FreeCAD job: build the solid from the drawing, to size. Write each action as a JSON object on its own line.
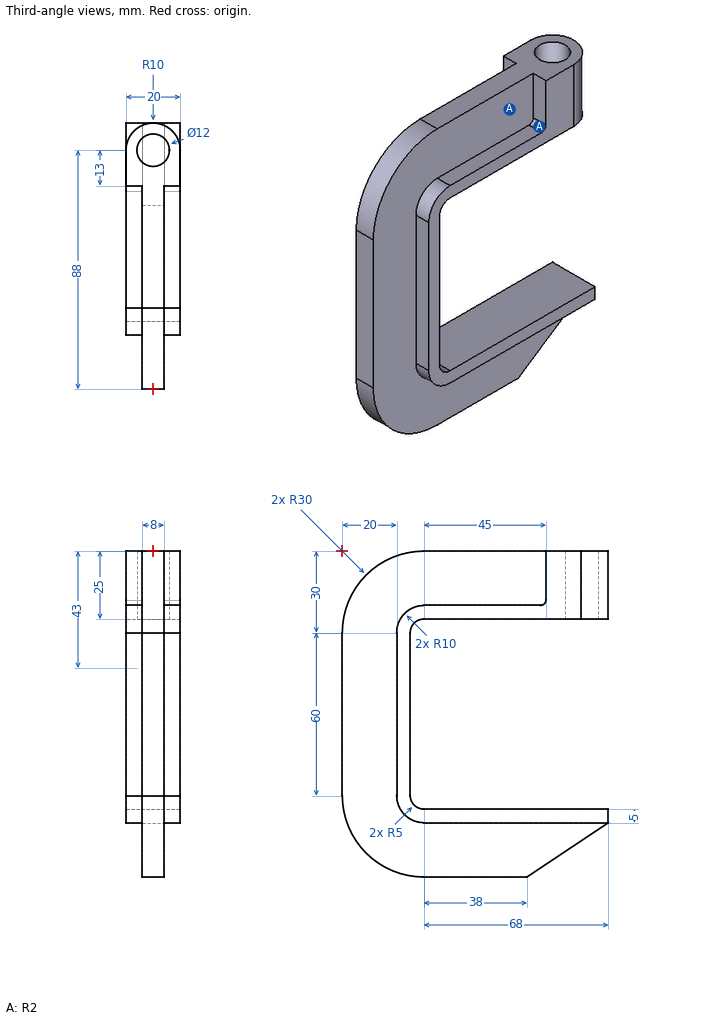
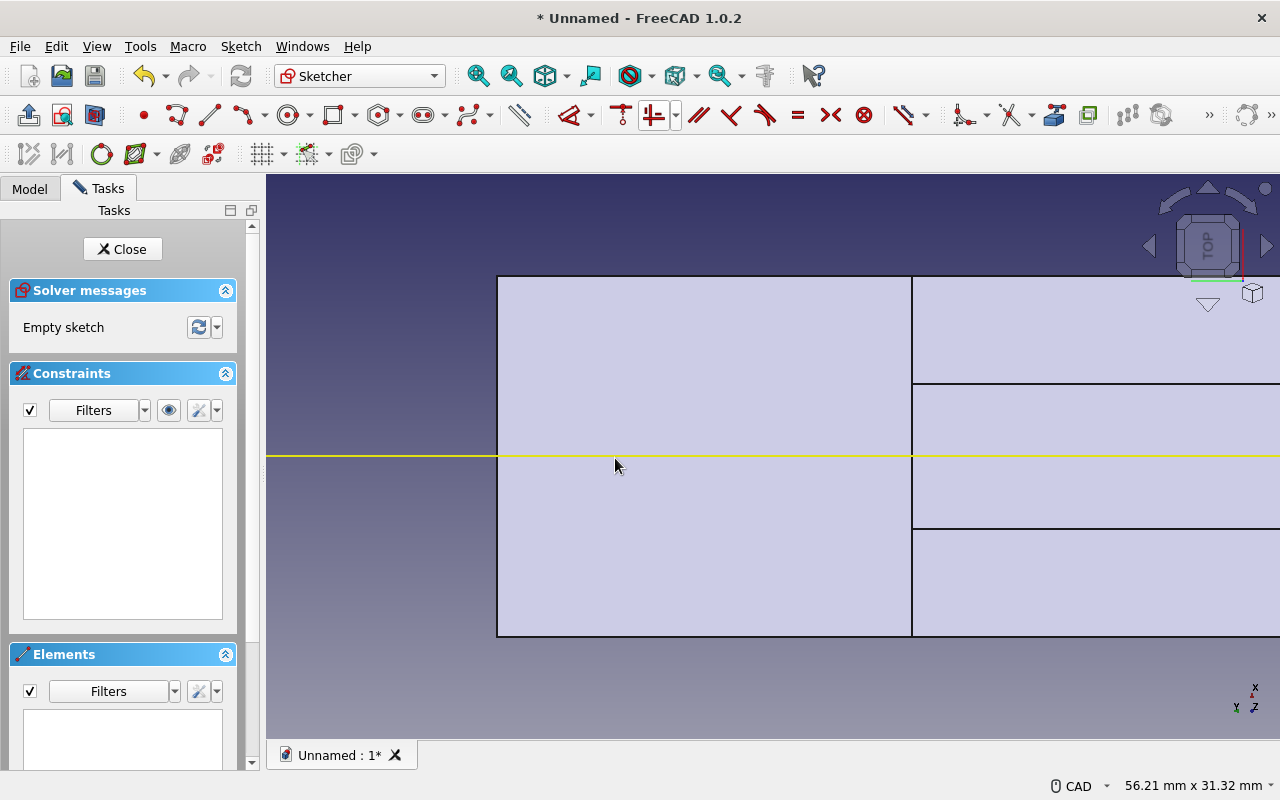
{"action": "key", "text": "g m"}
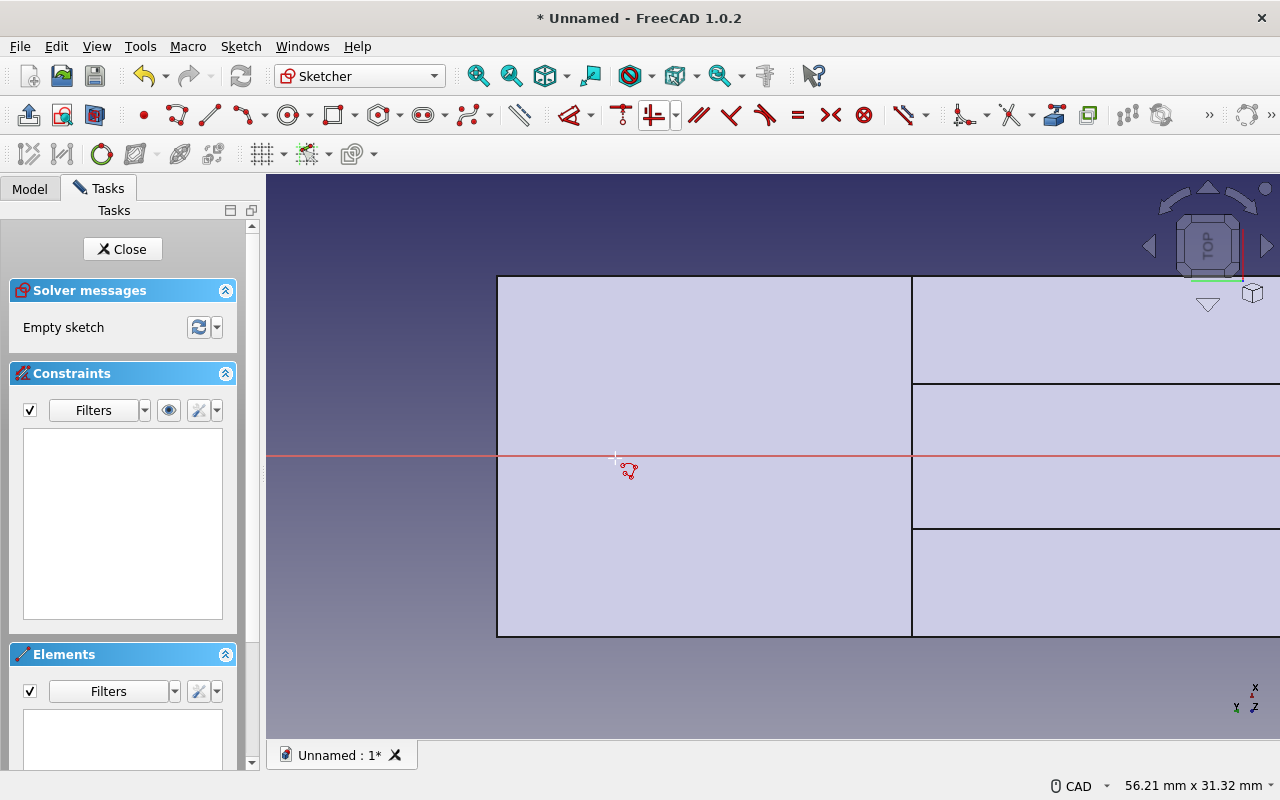
{"action": "left_click", "coordinate": [677, 637]}
{"action": "left_click", "coordinate": [912, 637]}
{"action": "left_click", "coordinate": [912, 276]}
{"action": "left_click", "coordinate": [677, 276]}
{"action": "right_click", "coordinate": [677, 276]}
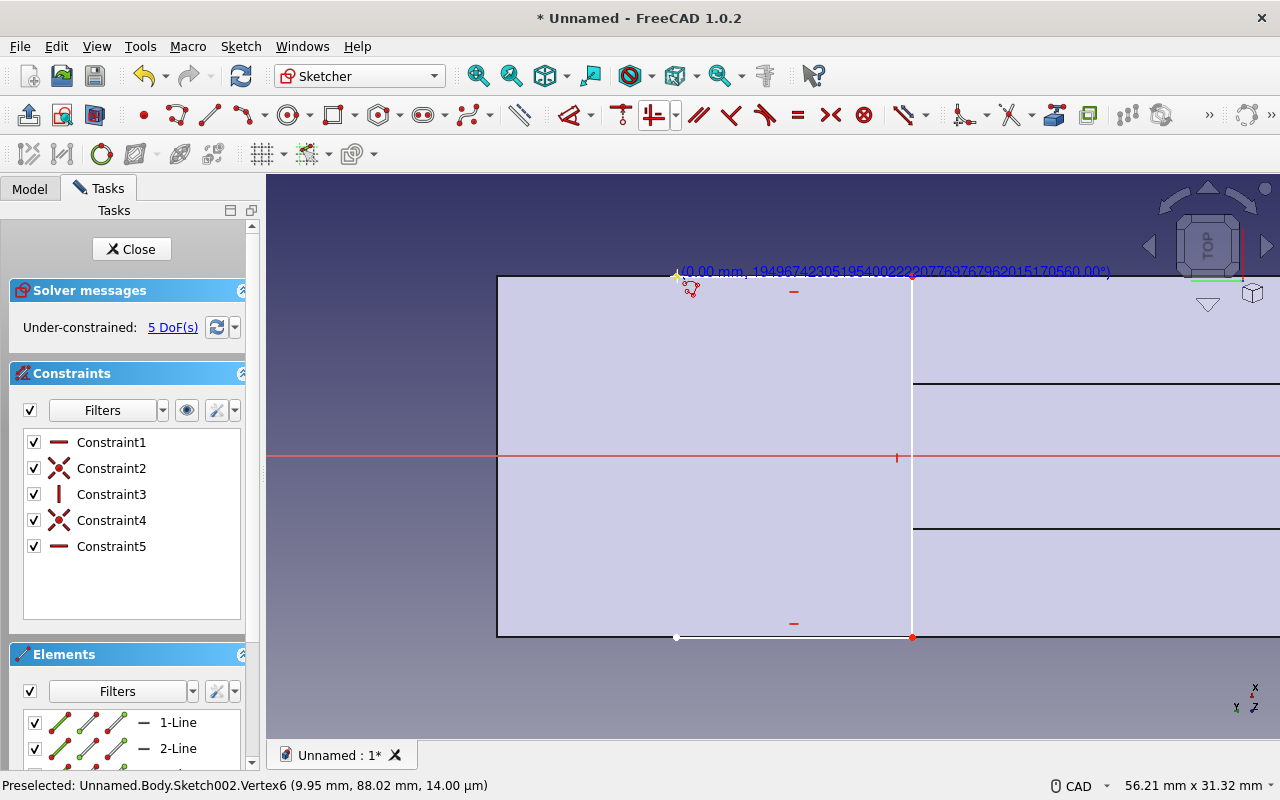
{"action": "key", "text": "g 3 a"}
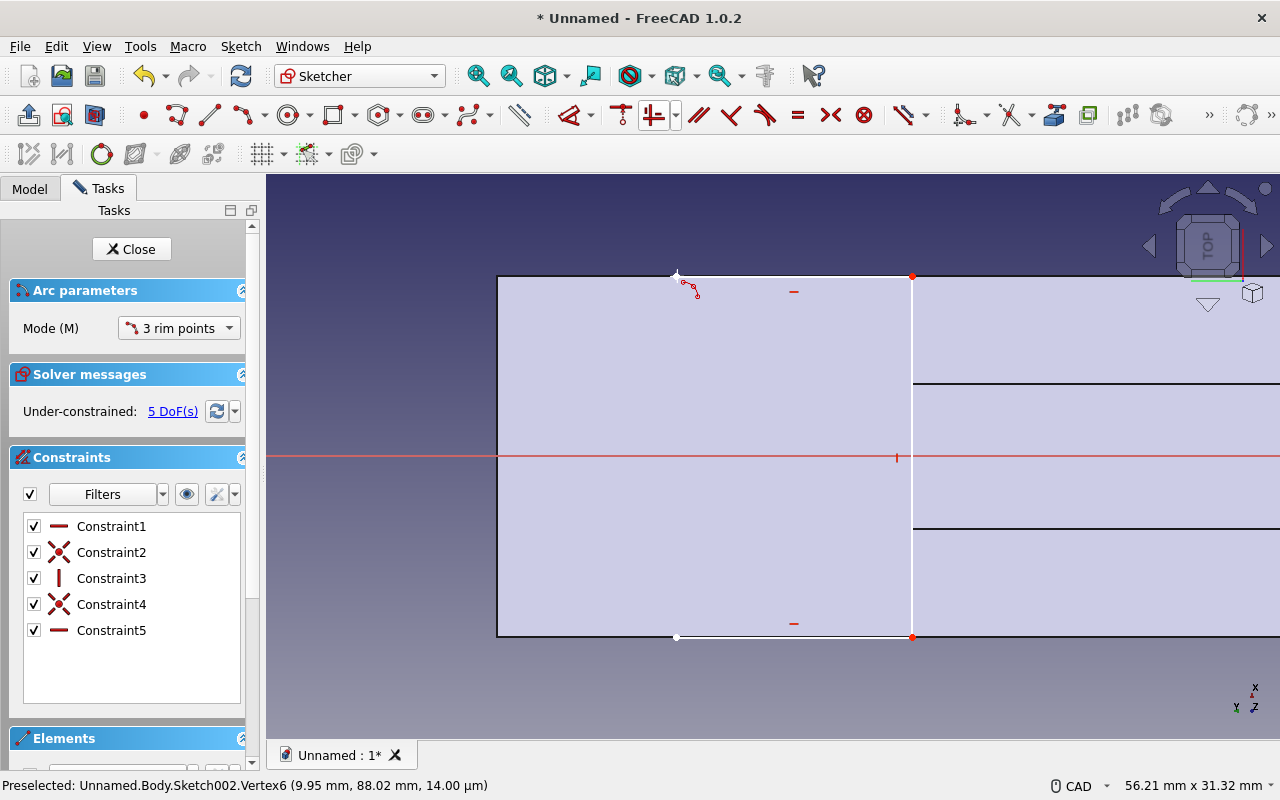
{"action": "left_click", "coordinate": [677, 277]}
{"action": "left_click", "coordinate": [677, 638]}
{"action": "left_click", "coordinate": [506, 401]}
{"action": "key", "text": "Escape"}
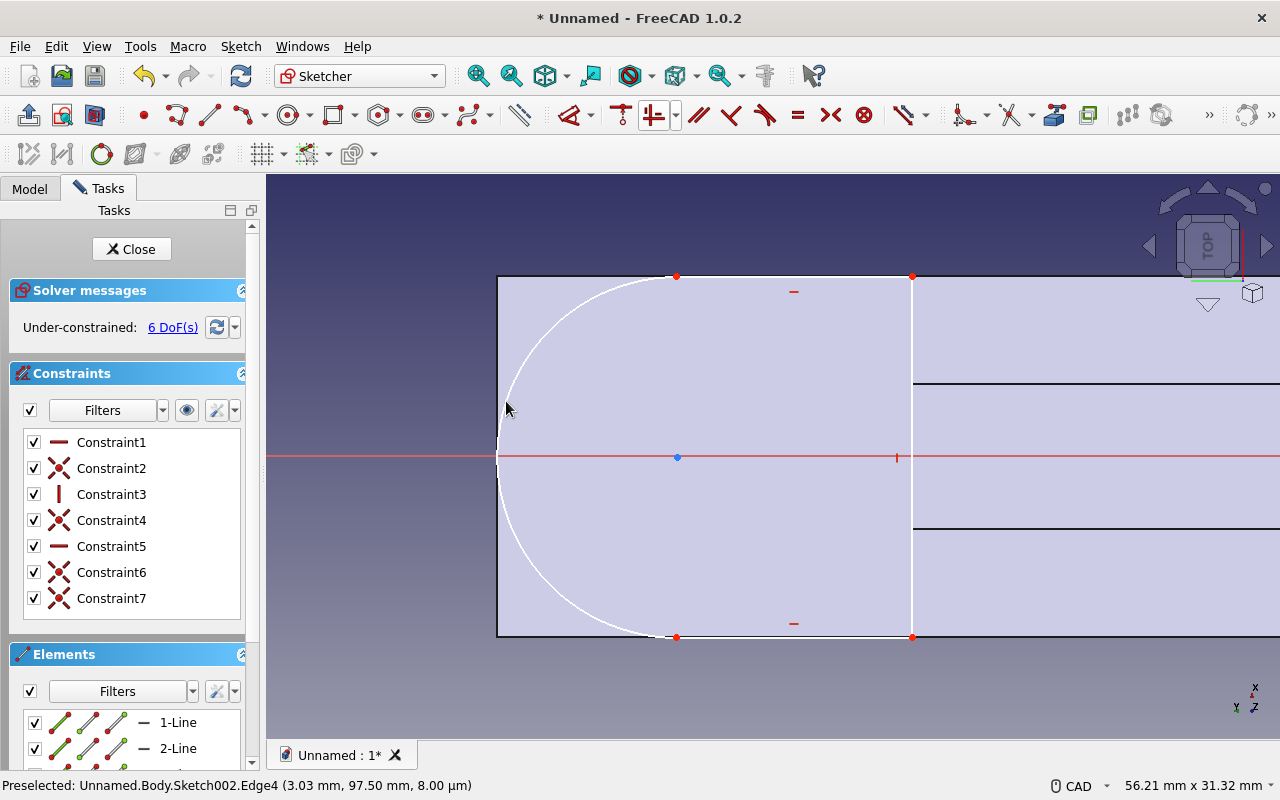
{"action": "left_click", "coordinate": [748, 638]}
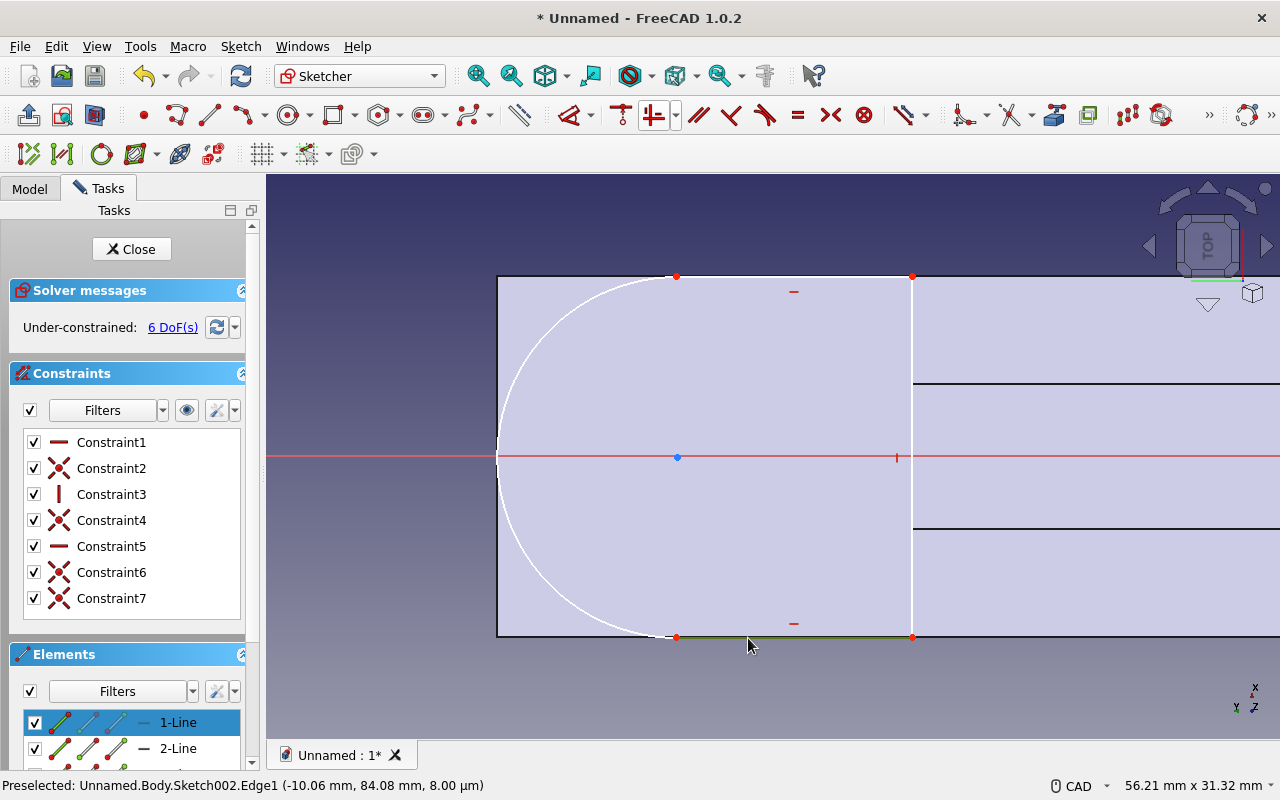
{"action": "left_click", "coordinate": [532, 352]}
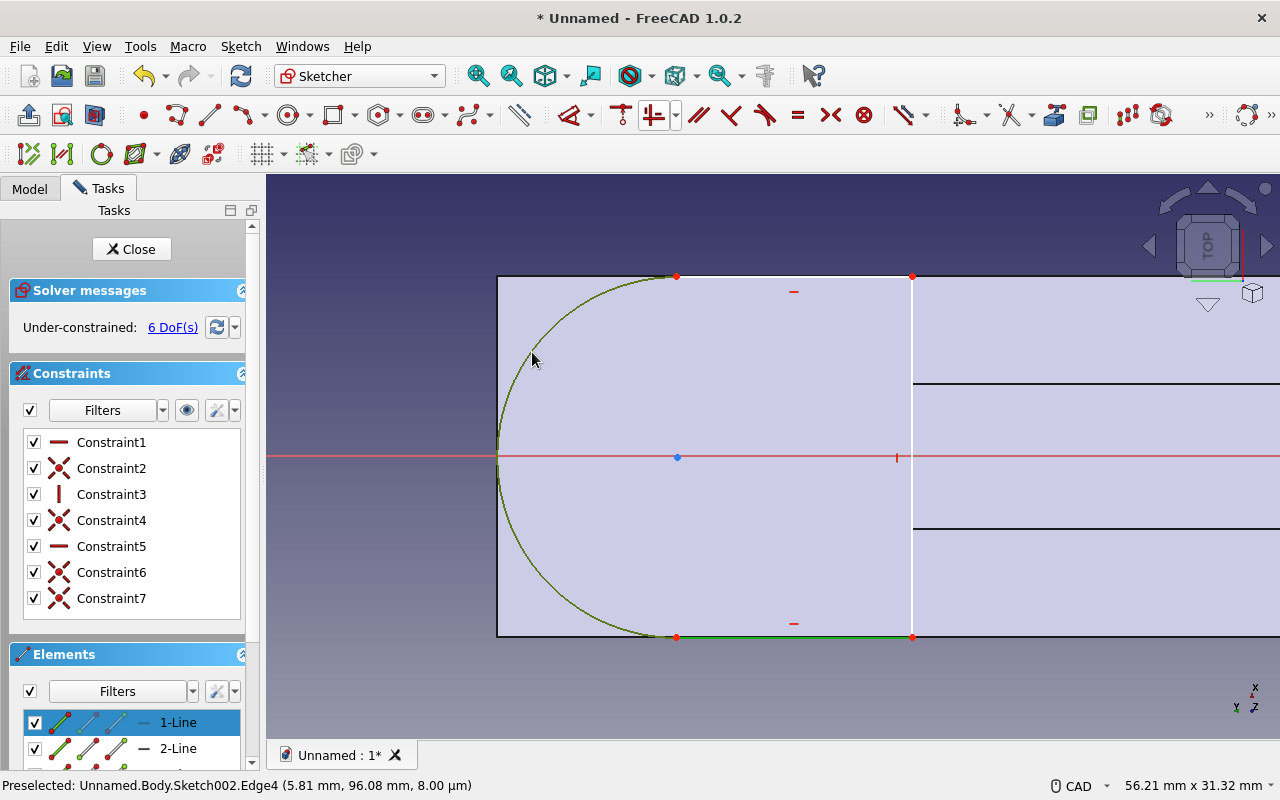
{"action": "key", "text": "t"}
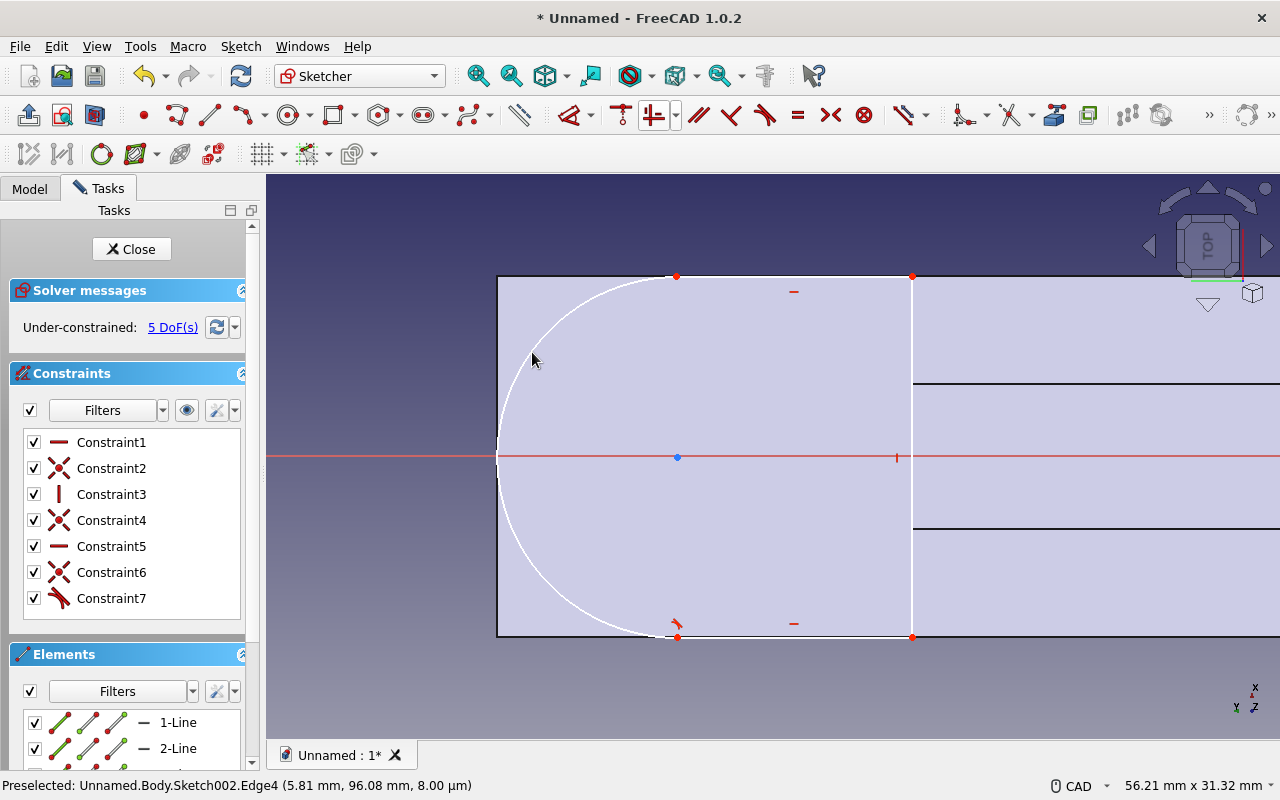
{"action": "left_click", "coordinate": [842, 277]}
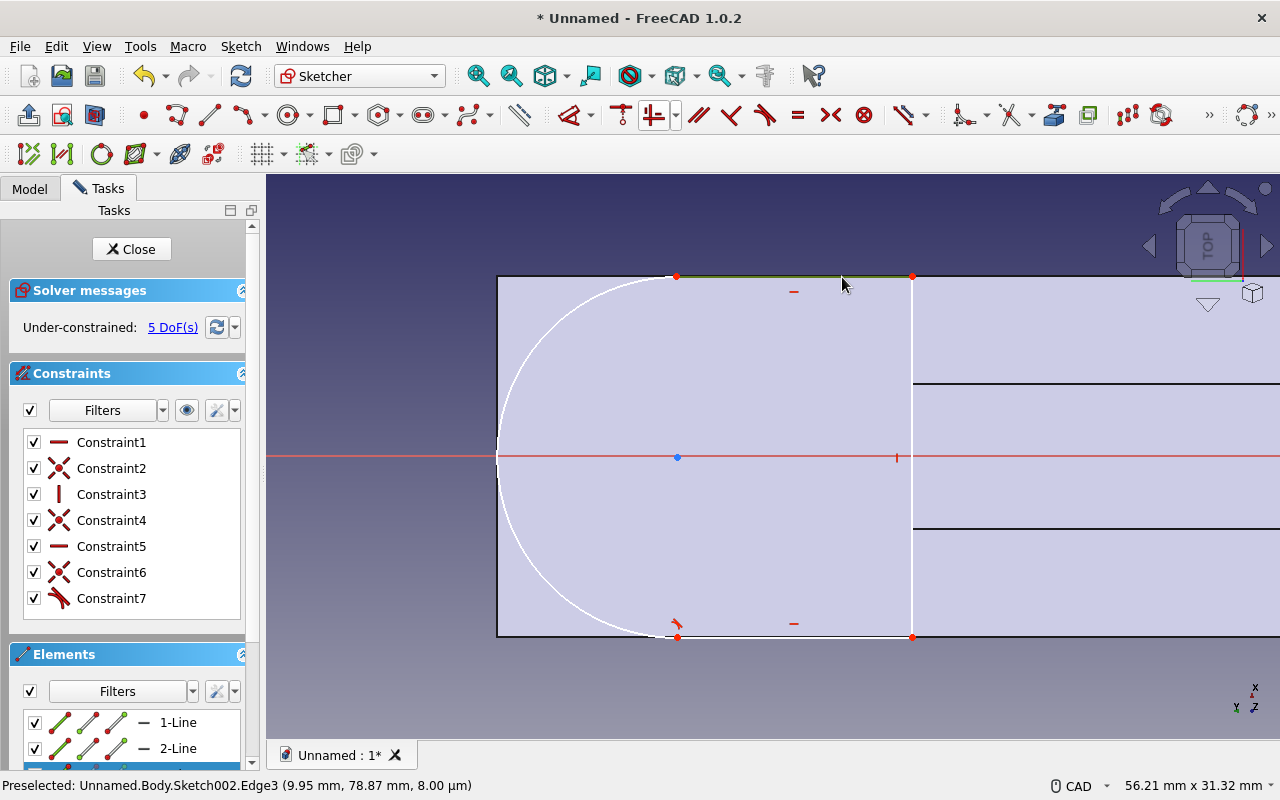
{"action": "left_click", "coordinate": [531, 352]}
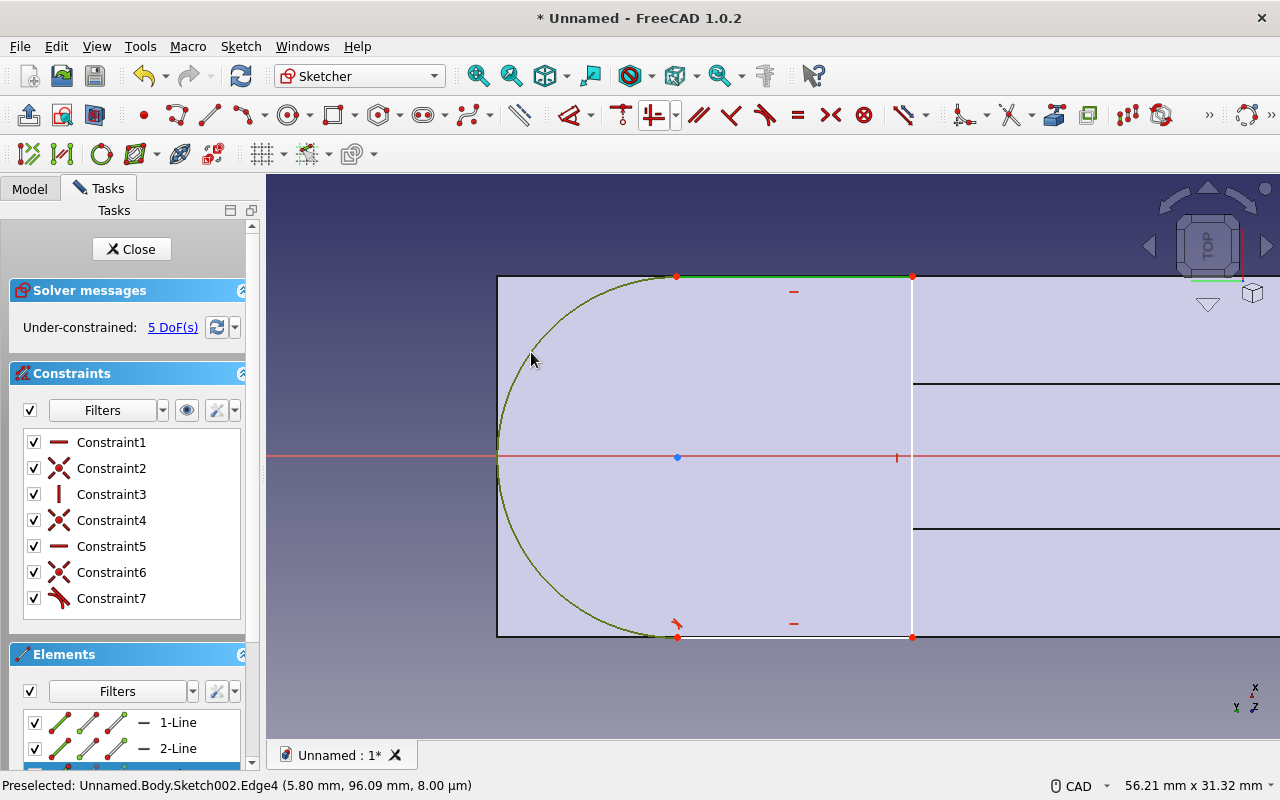
{"action": "key", "text": "t"}